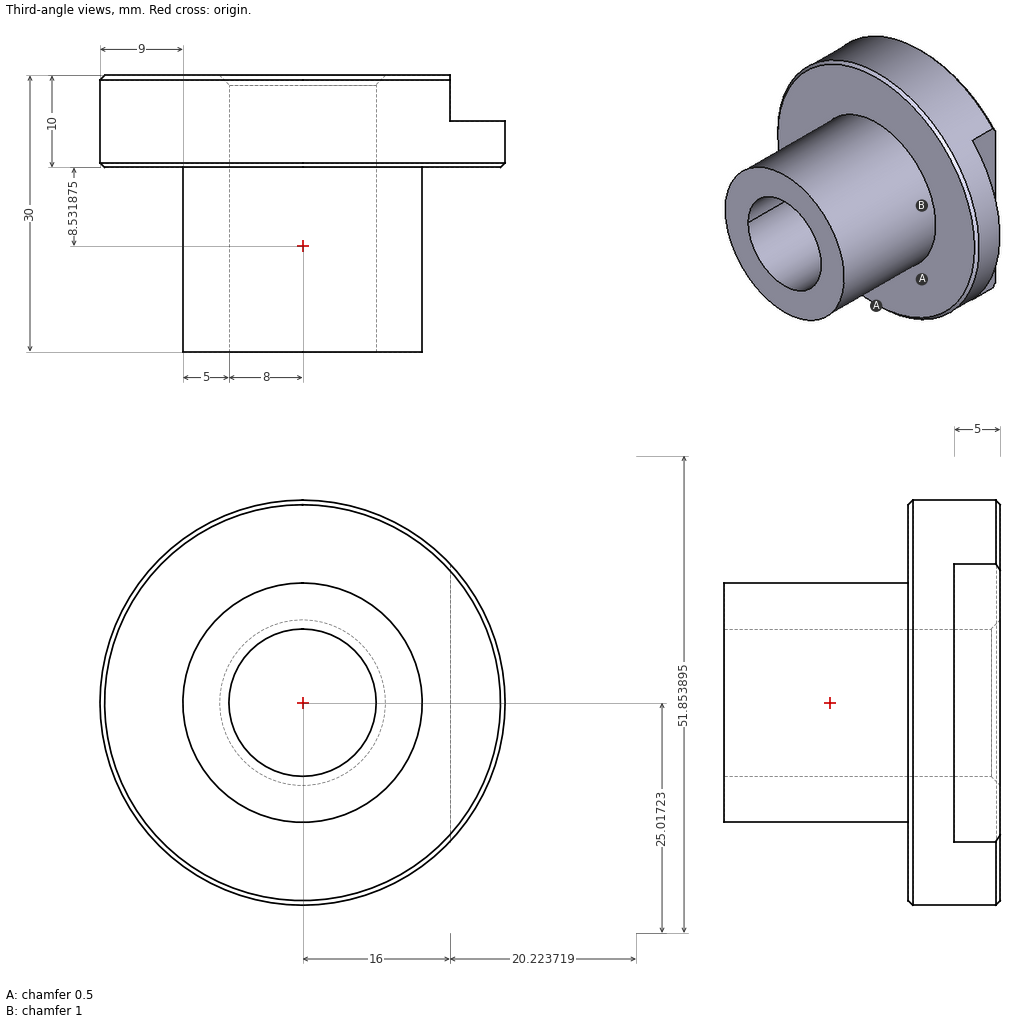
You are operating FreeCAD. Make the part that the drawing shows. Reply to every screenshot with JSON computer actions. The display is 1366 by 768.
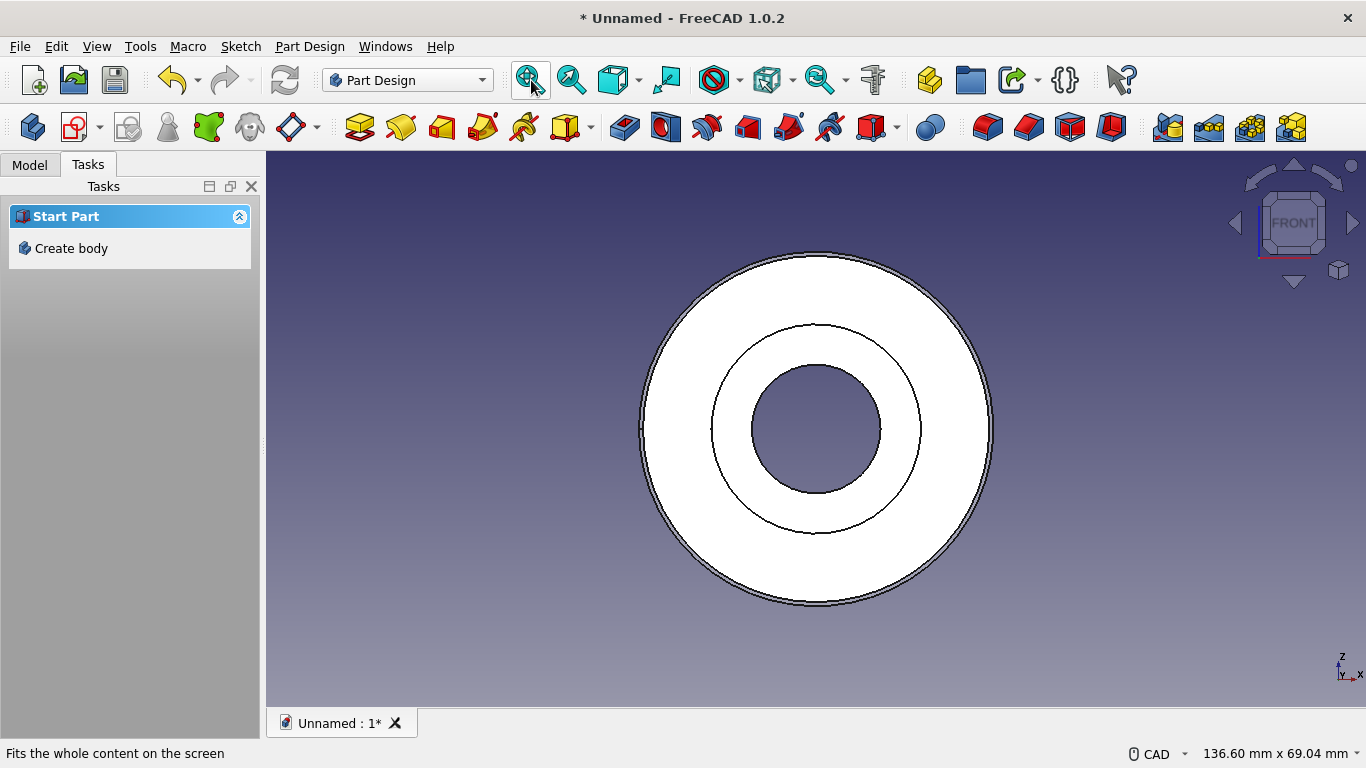
{"action": "key", "text": "3"}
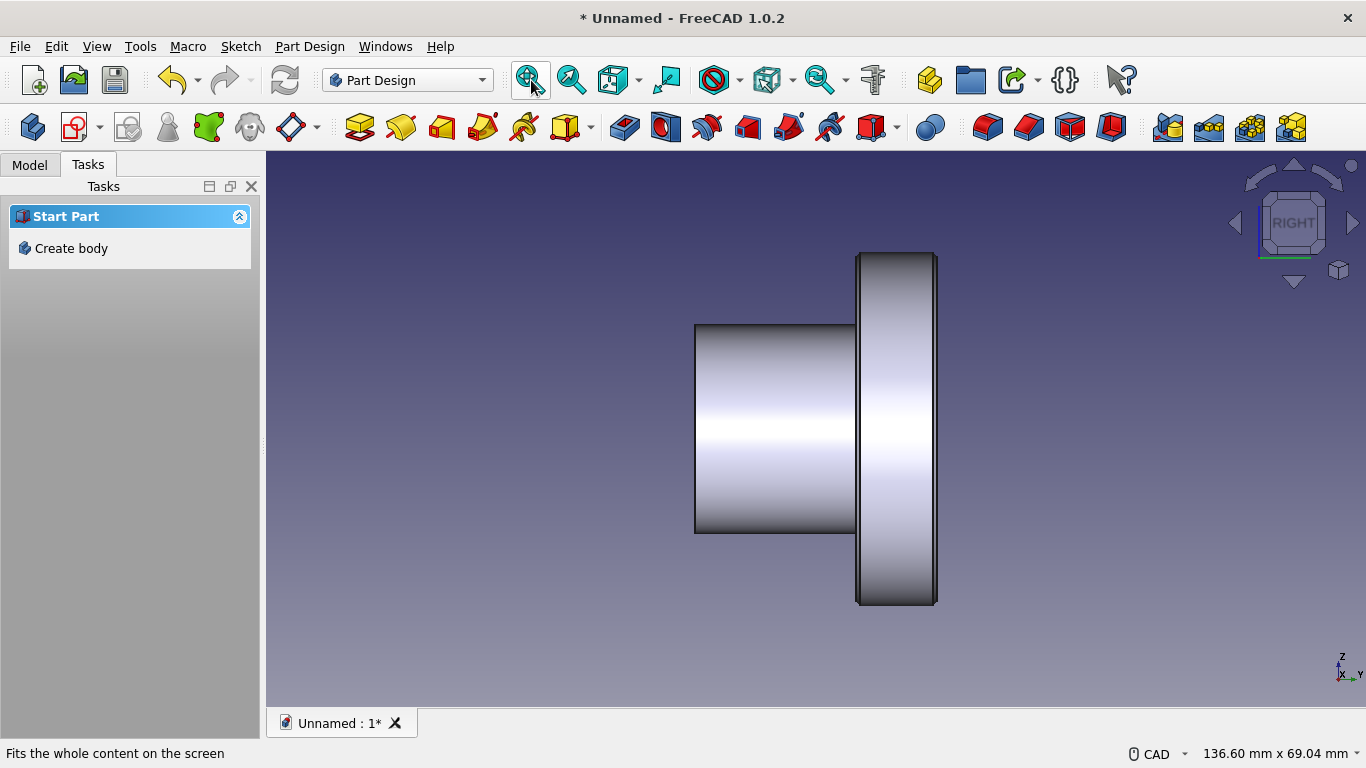
{"action": "key", "text": "5"}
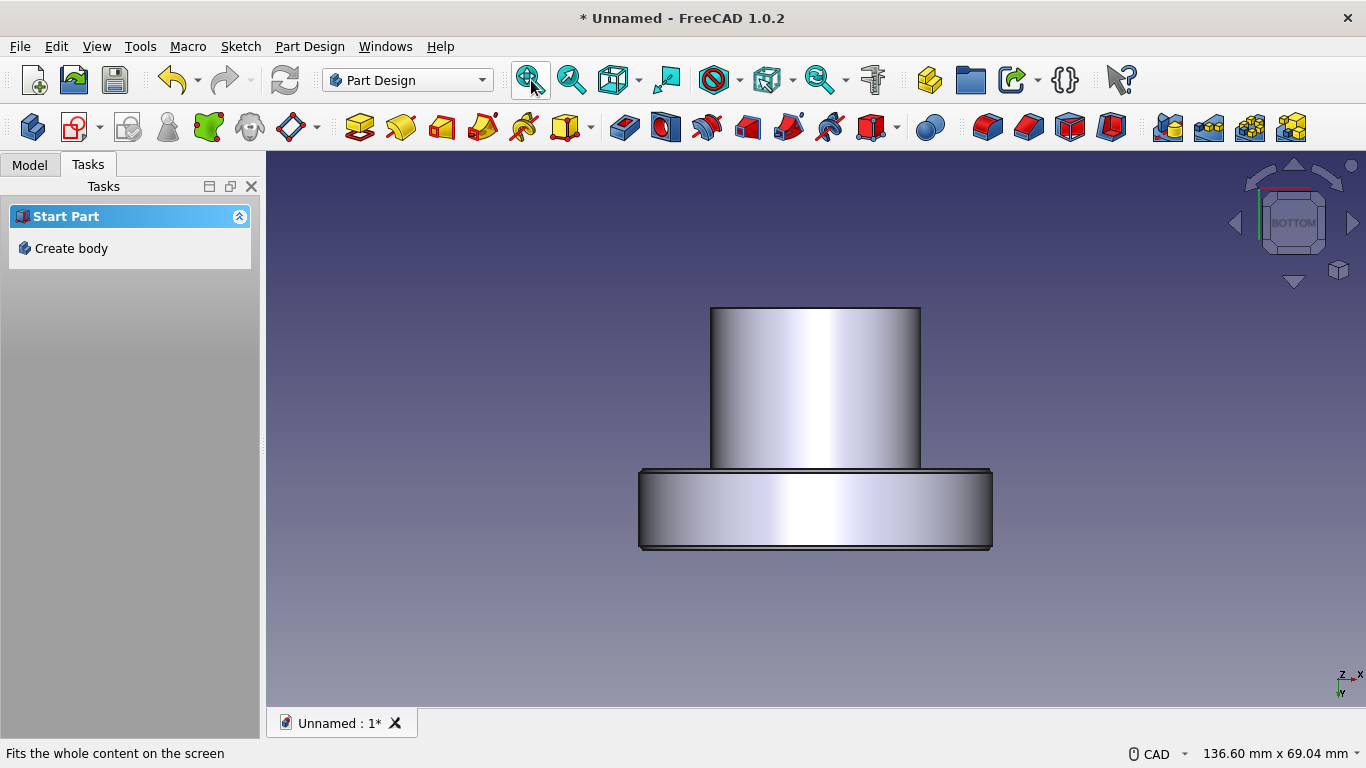
{"action": "left_click", "coordinate": [531, 80]}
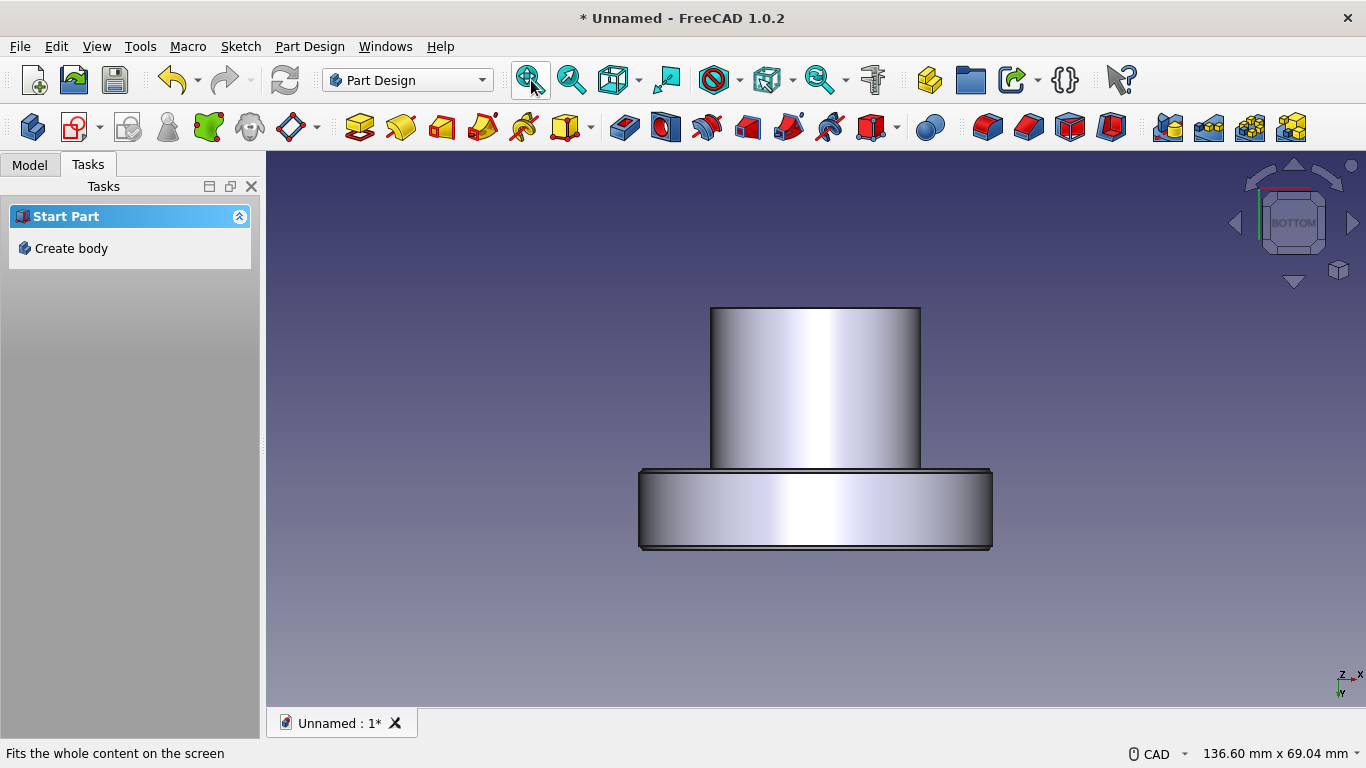
{"action": "key", "text": "4"}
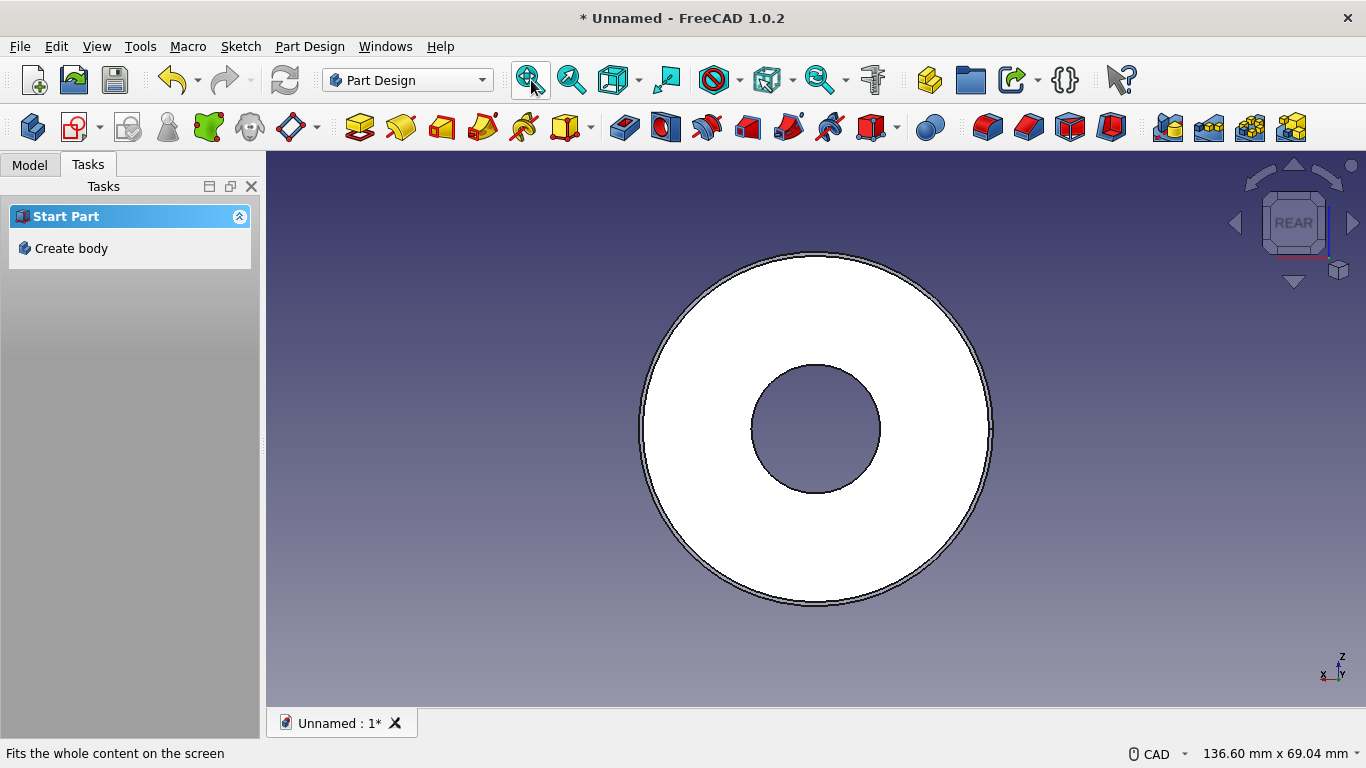
{"action": "left_click", "coordinate": [751, 428]}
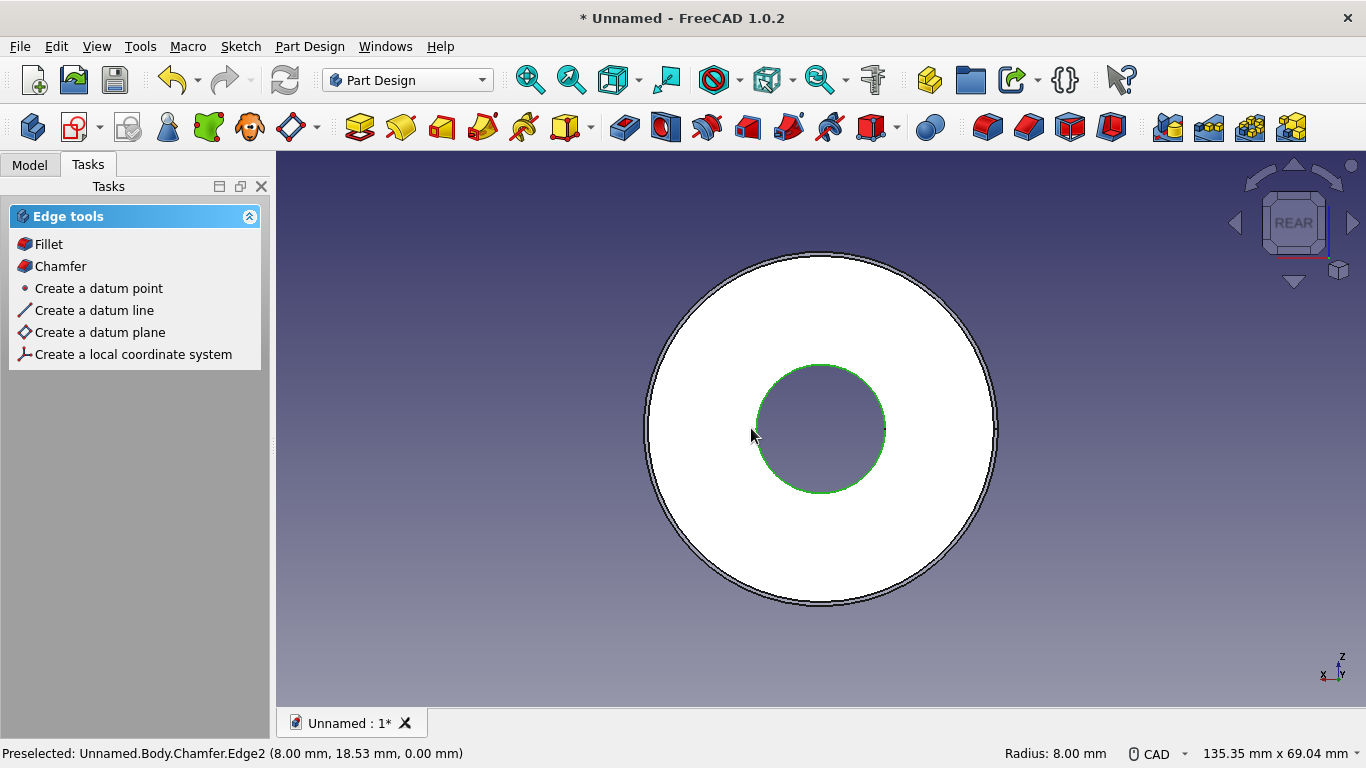
{"action": "left_click", "coordinate": [1029, 128]}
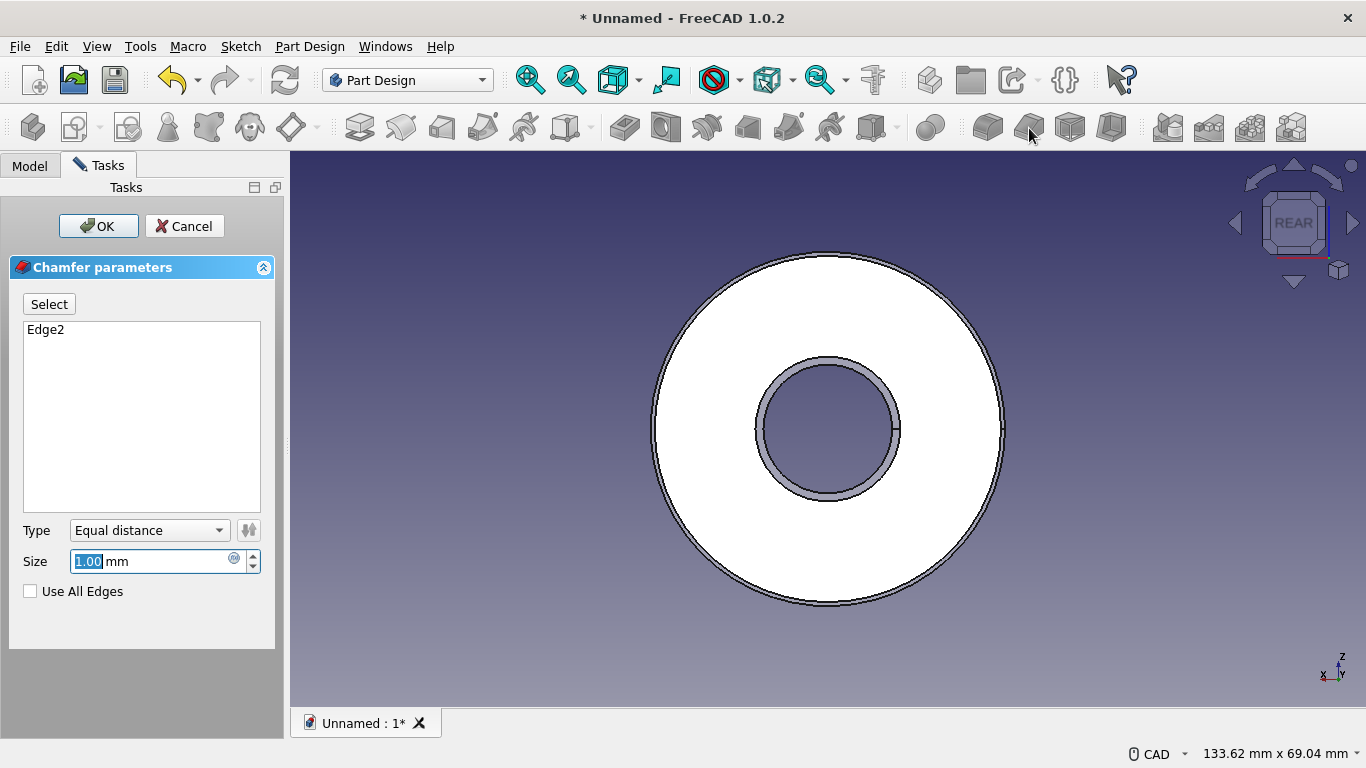
{"action": "type", "text": "1"}
{"action": "key", "text": "Tab"}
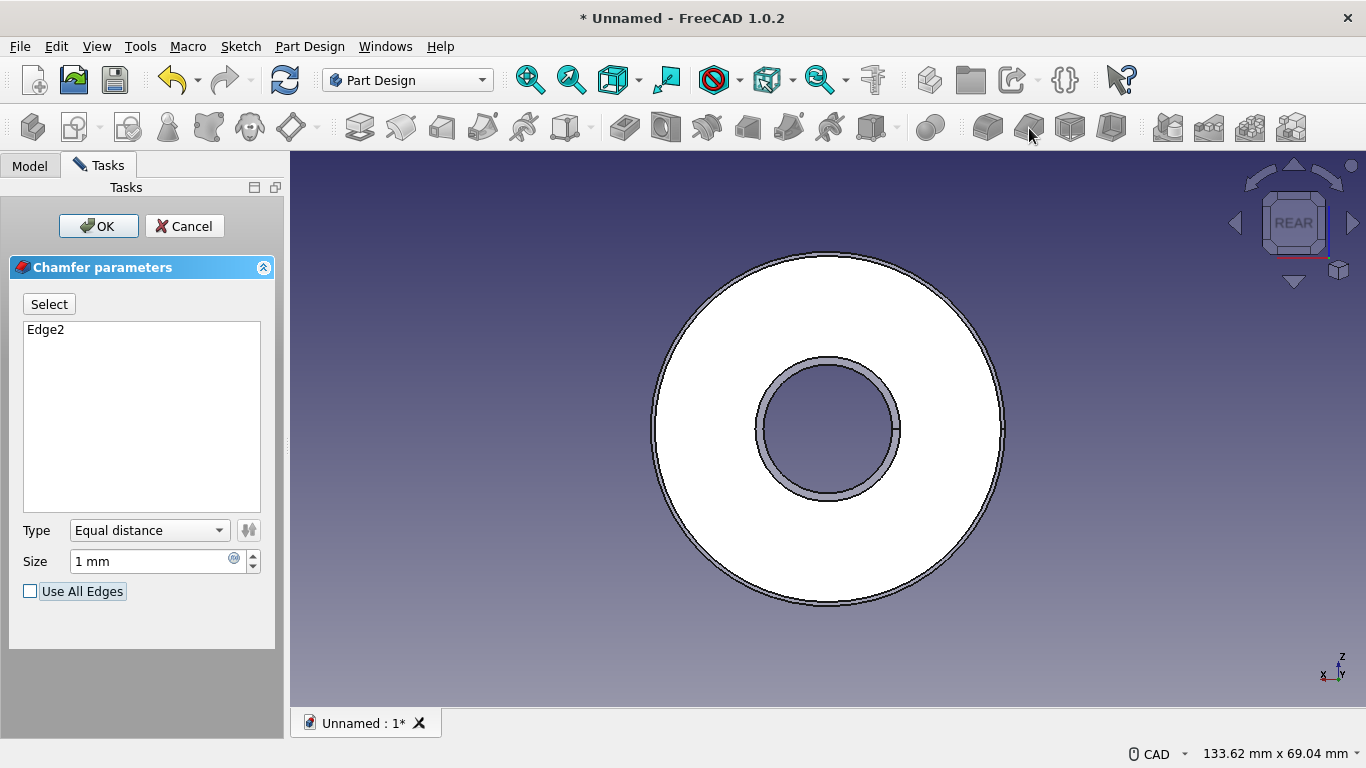
{"action": "left_click", "coordinate": [99, 226]}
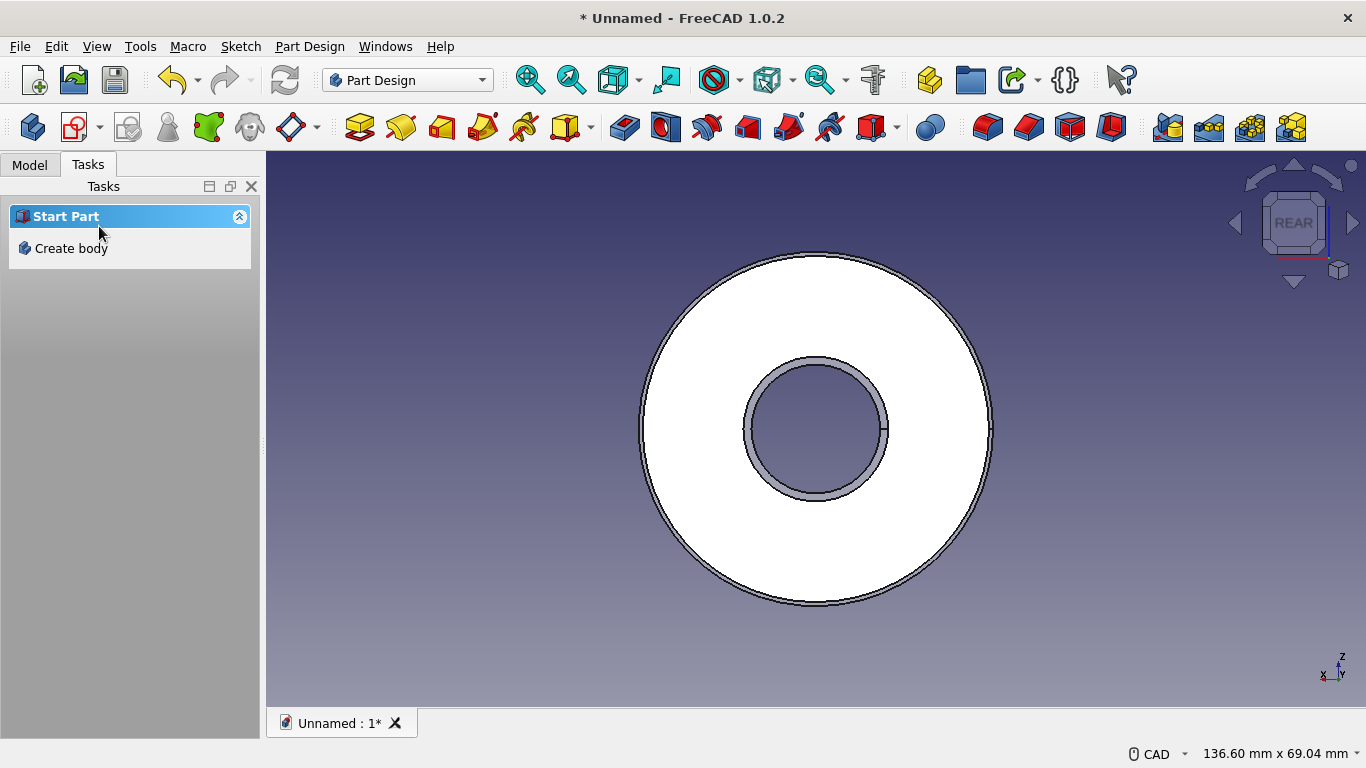
{"action": "left_click", "coordinate": [766, 329]}